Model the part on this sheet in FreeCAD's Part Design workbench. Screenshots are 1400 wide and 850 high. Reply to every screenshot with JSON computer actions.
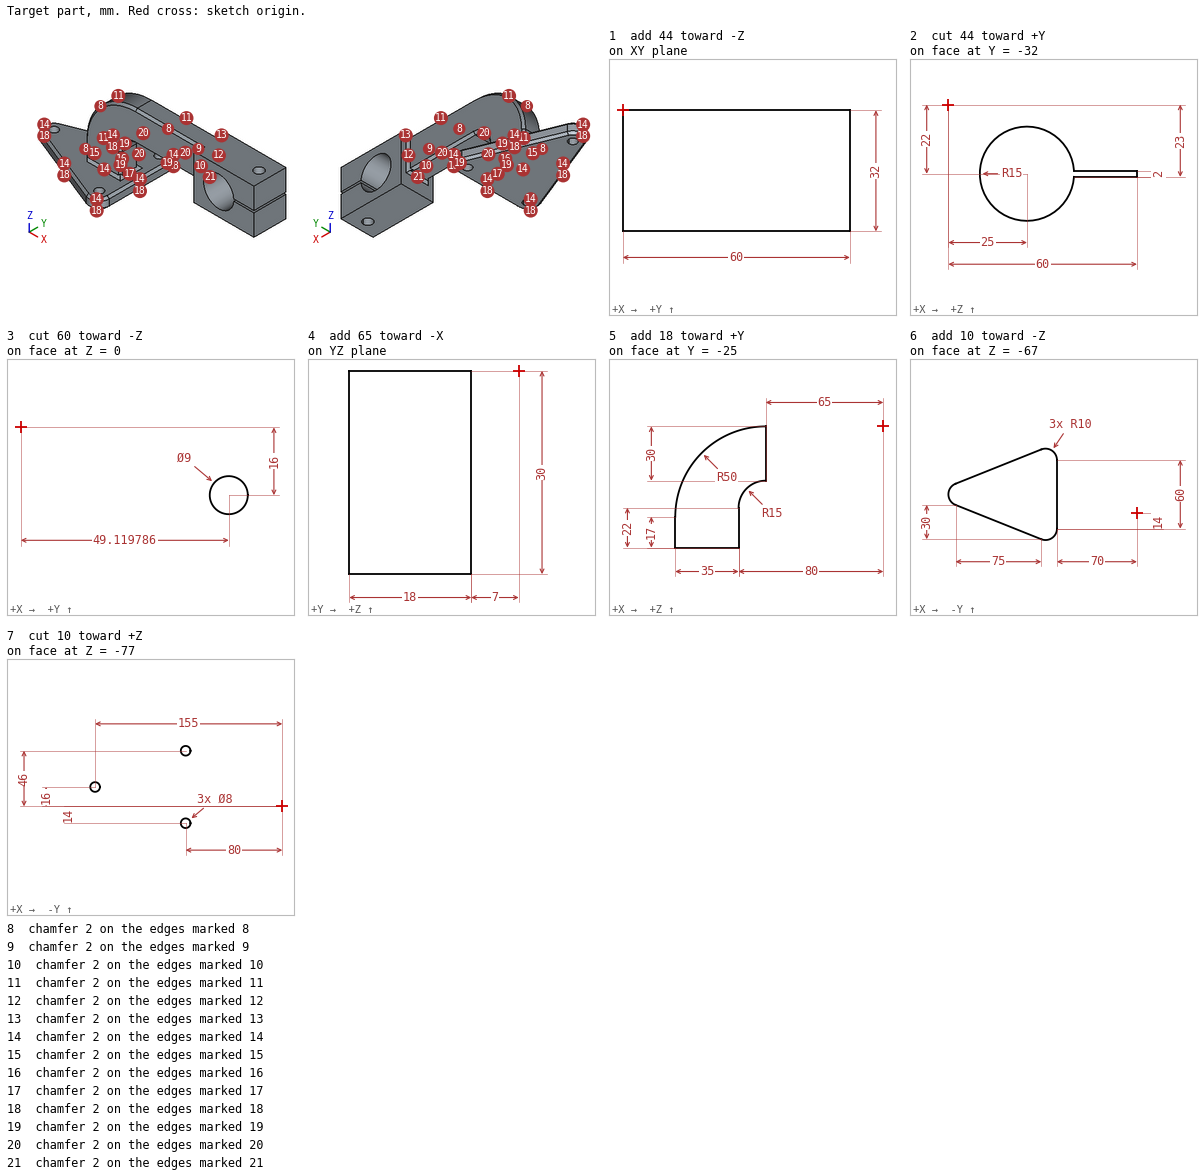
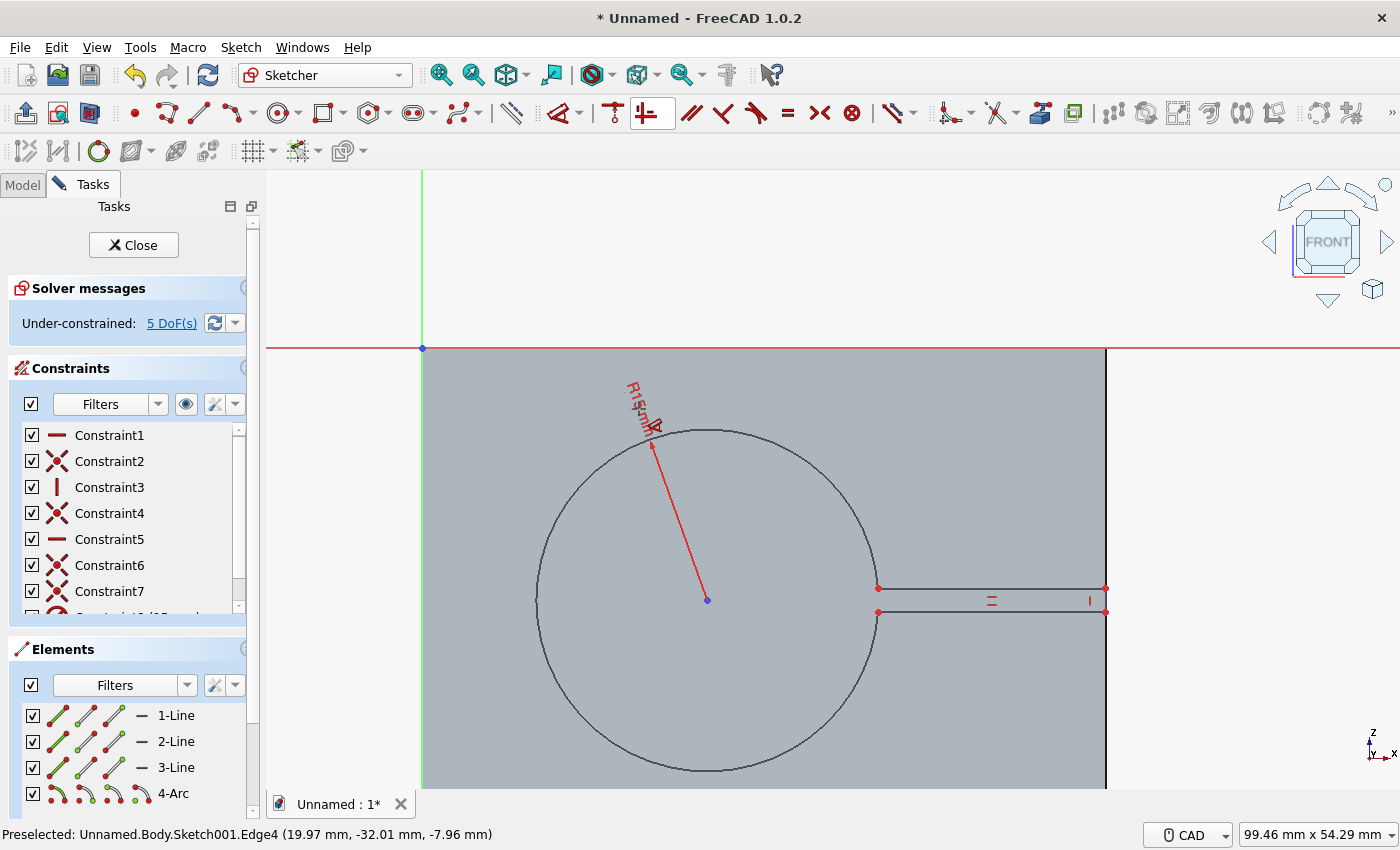
{"action": "scroll", "coordinate": [1106, 603], "scroll_direction": "up", "scroll_amount": 3}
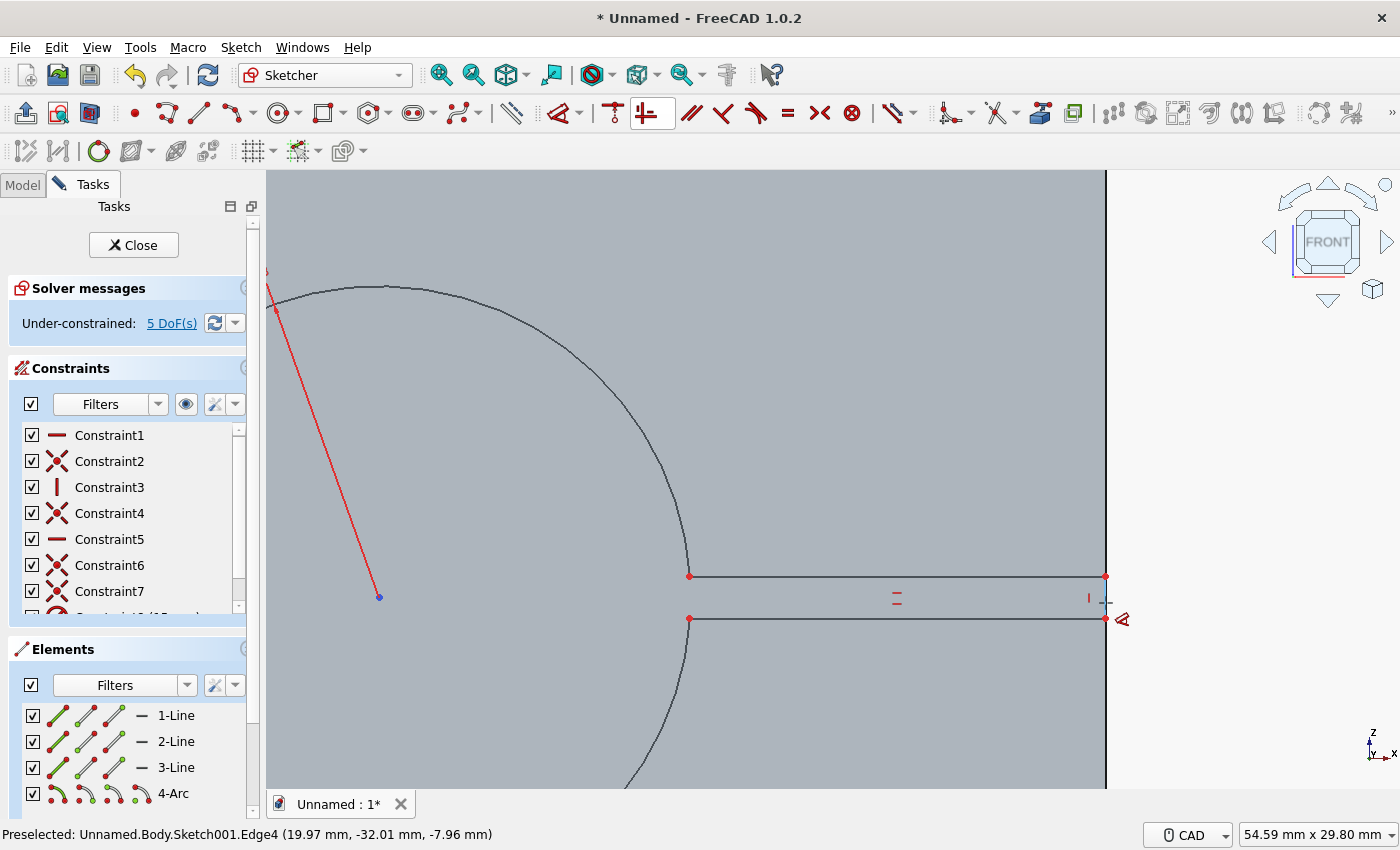
{"action": "left_click", "coordinate": [1105, 602]}
{"action": "left_click", "coordinate": [1139, 598]}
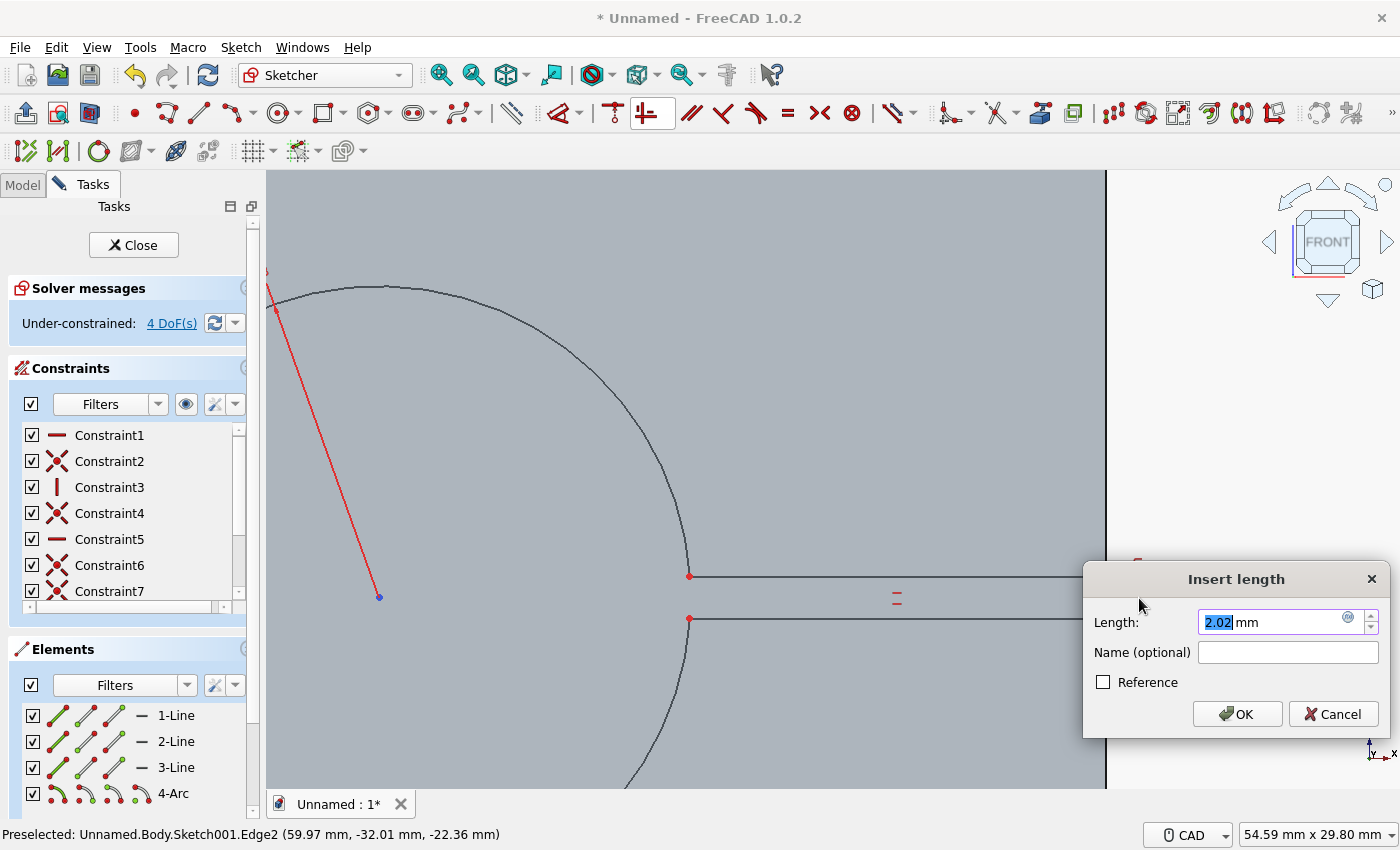
{"action": "type", "text": "2"}
{"action": "key", "text": "Return"}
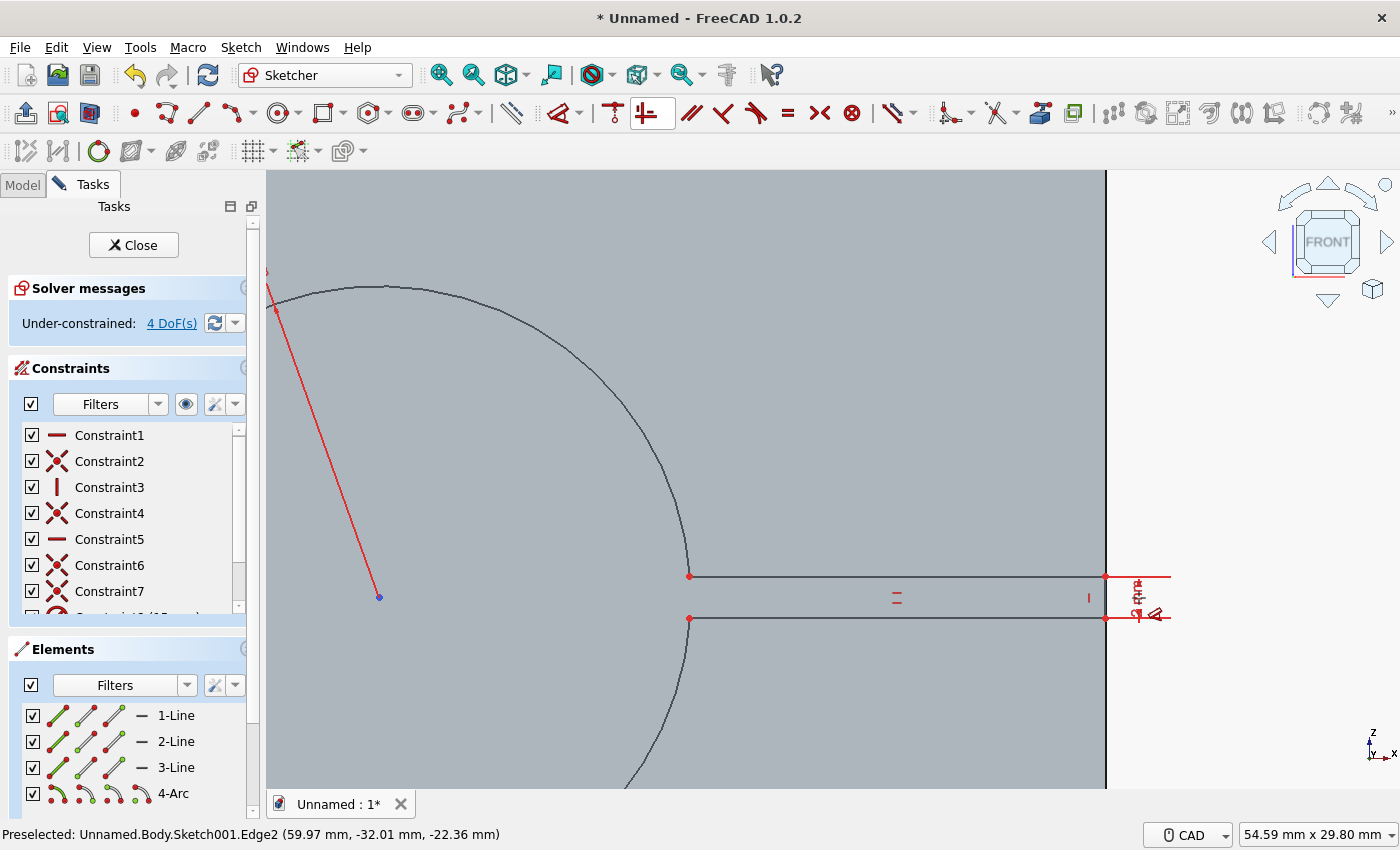
{"action": "left_click", "coordinate": [690, 618]}
{"action": "left_click", "coordinate": [724, 408]}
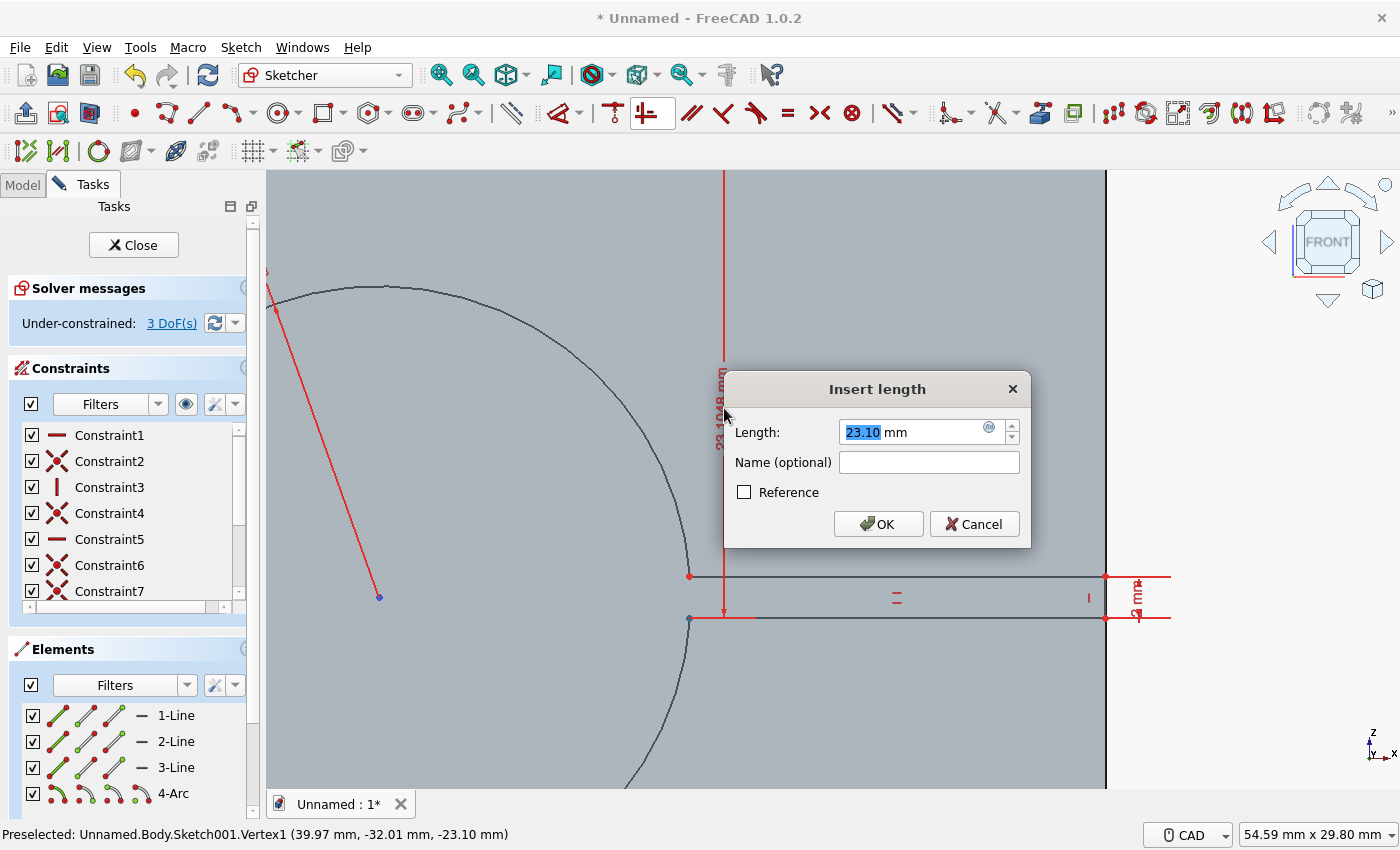
{"action": "type", "text": "23"}
{"action": "key", "text": "Return"}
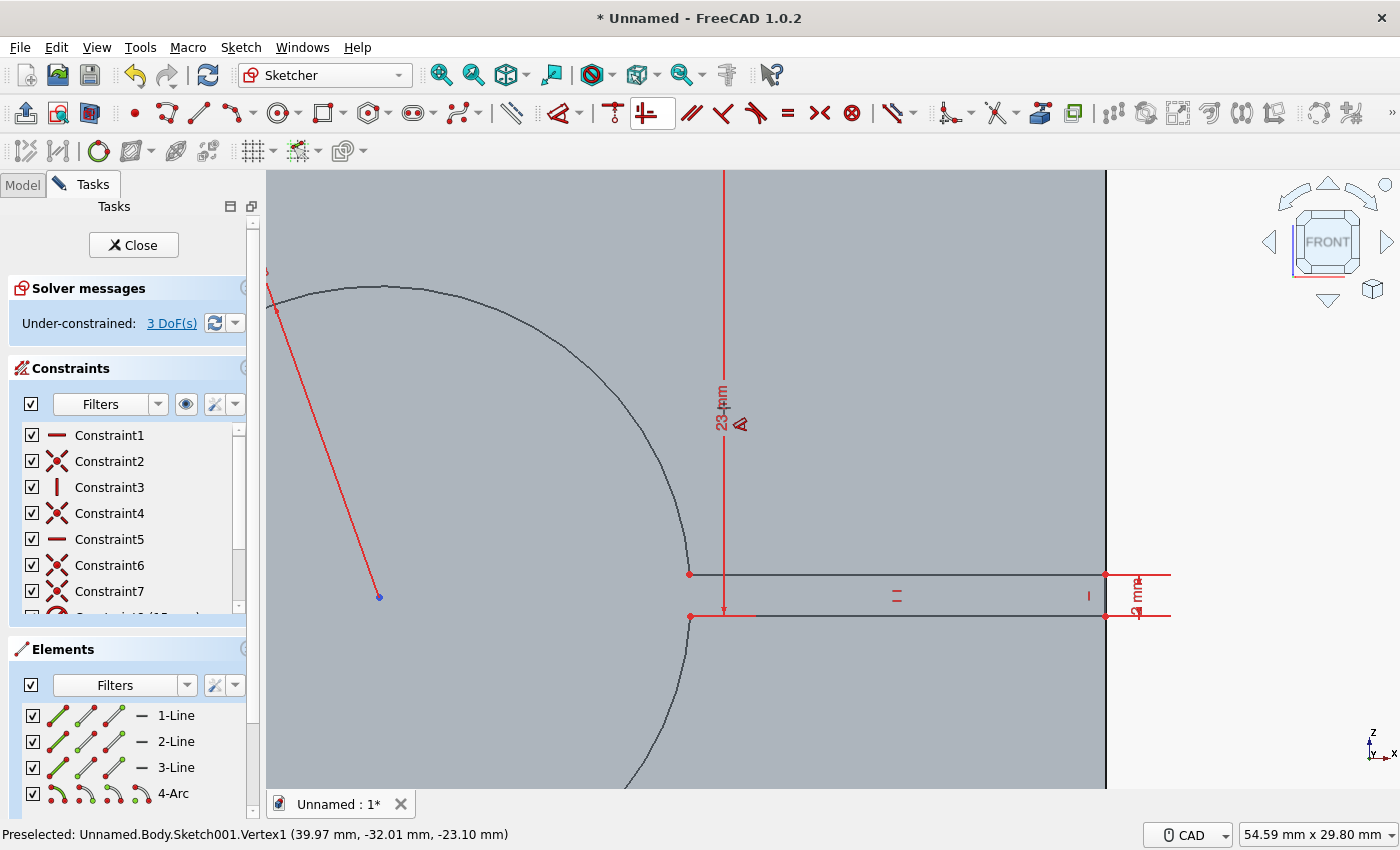
{"action": "left_click", "coordinate": [1105, 616]}
{"action": "left_click", "coordinate": [700, 650]}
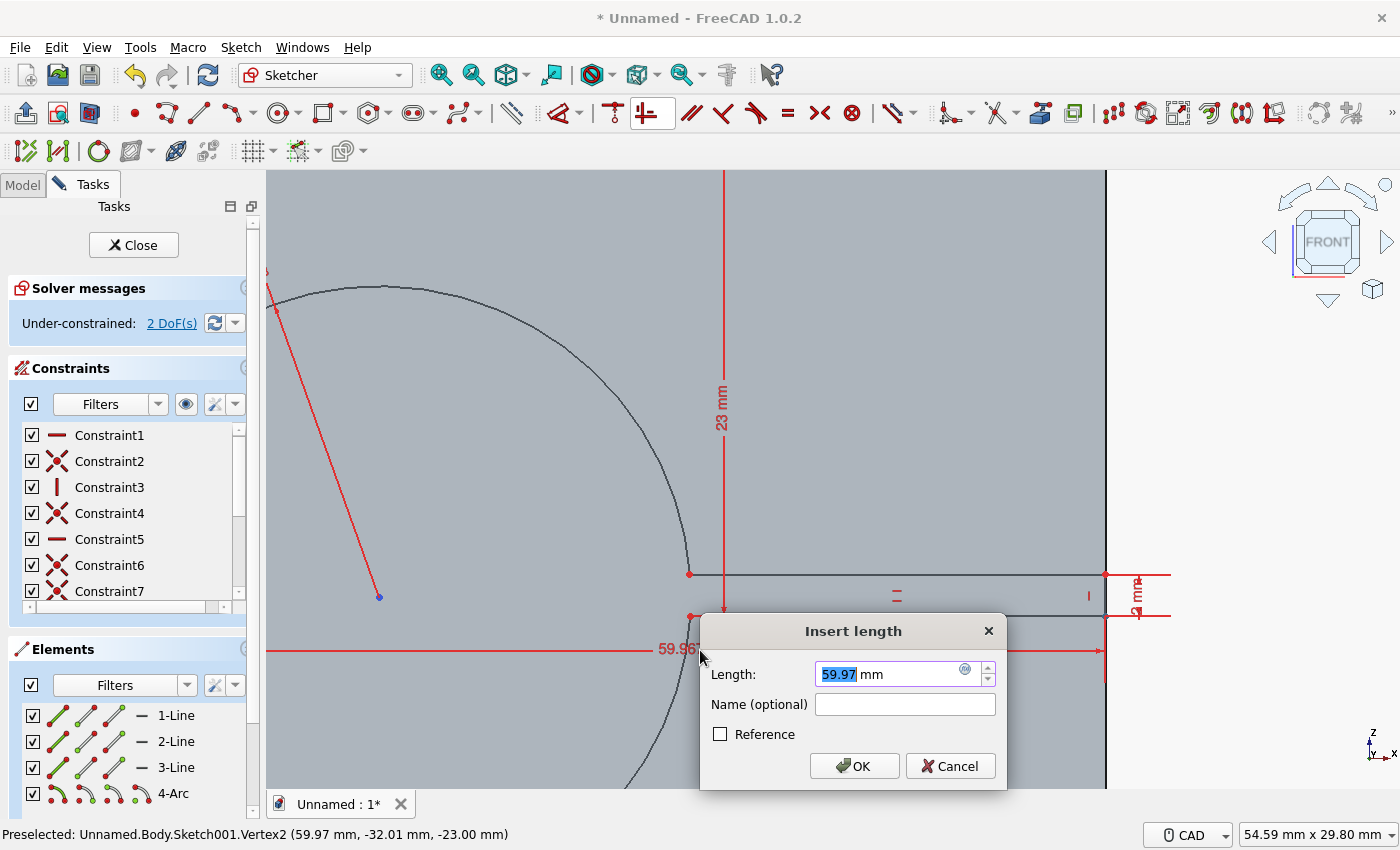
{"action": "type", "text": "60"}
{"action": "key", "text": "Return"}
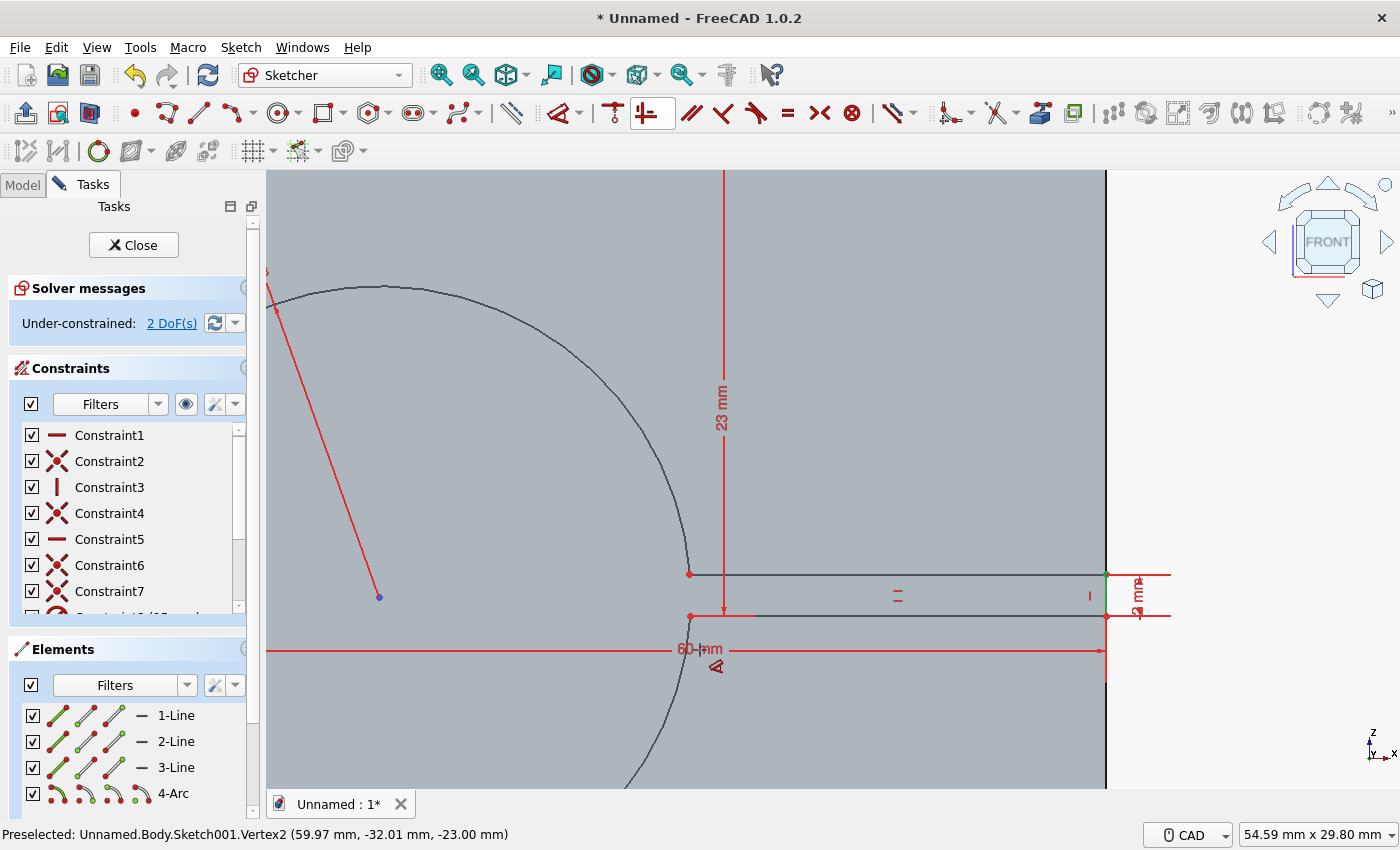
{"action": "left_click", "coordinate": [379, 598]}
{"action": "left_click", "coordinate": [337, 632]}